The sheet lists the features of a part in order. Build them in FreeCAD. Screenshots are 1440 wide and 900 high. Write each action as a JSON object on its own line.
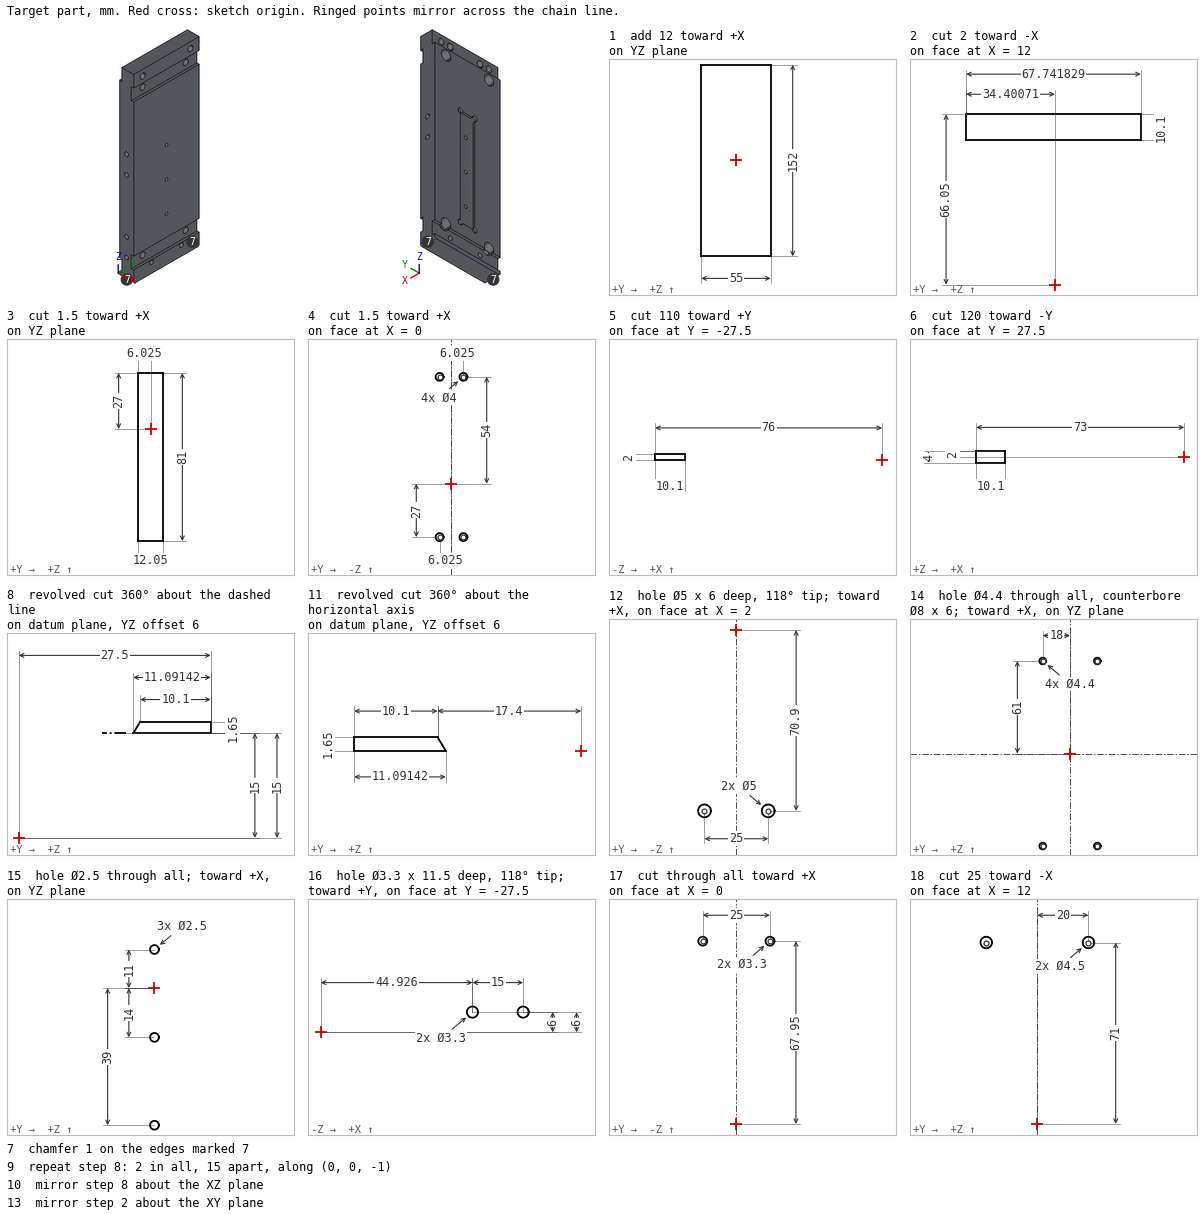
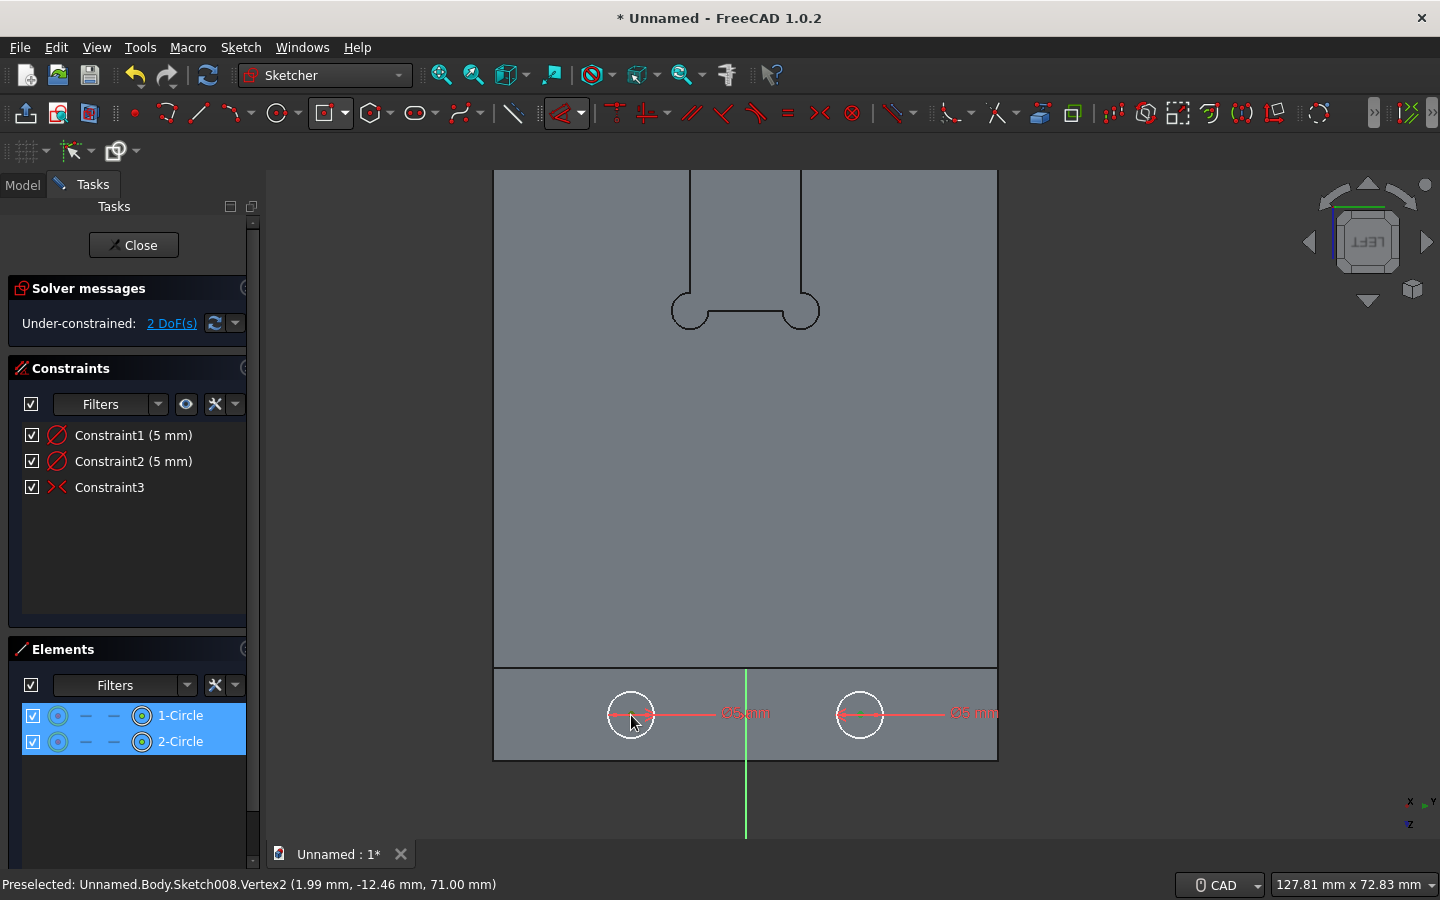
{"action": "key", "text": "l"}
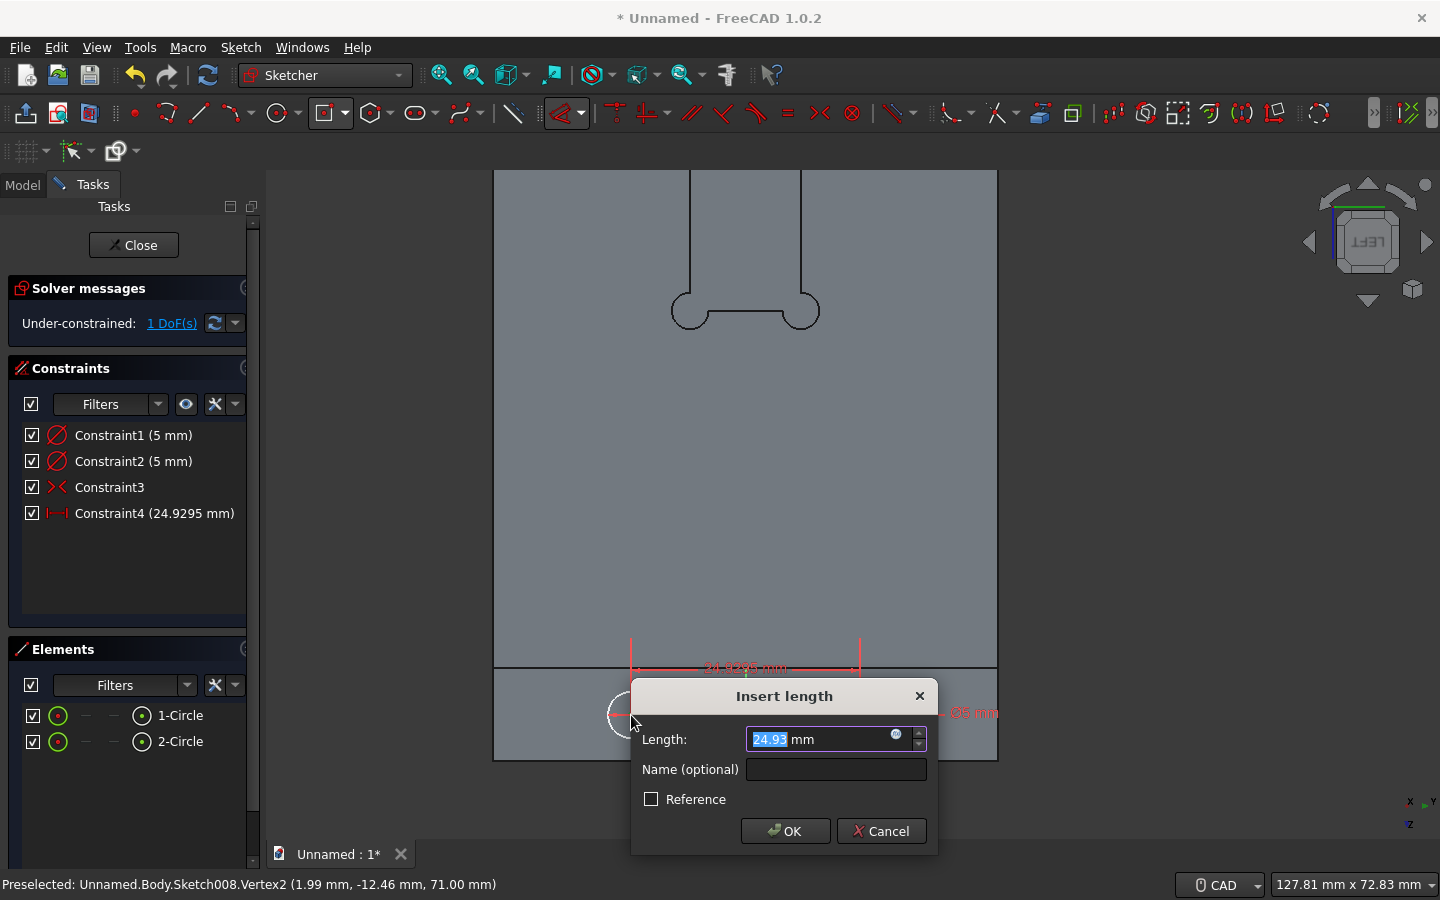
{"action": "type", "text": "25"}
{"action": "key", "text": "Return"}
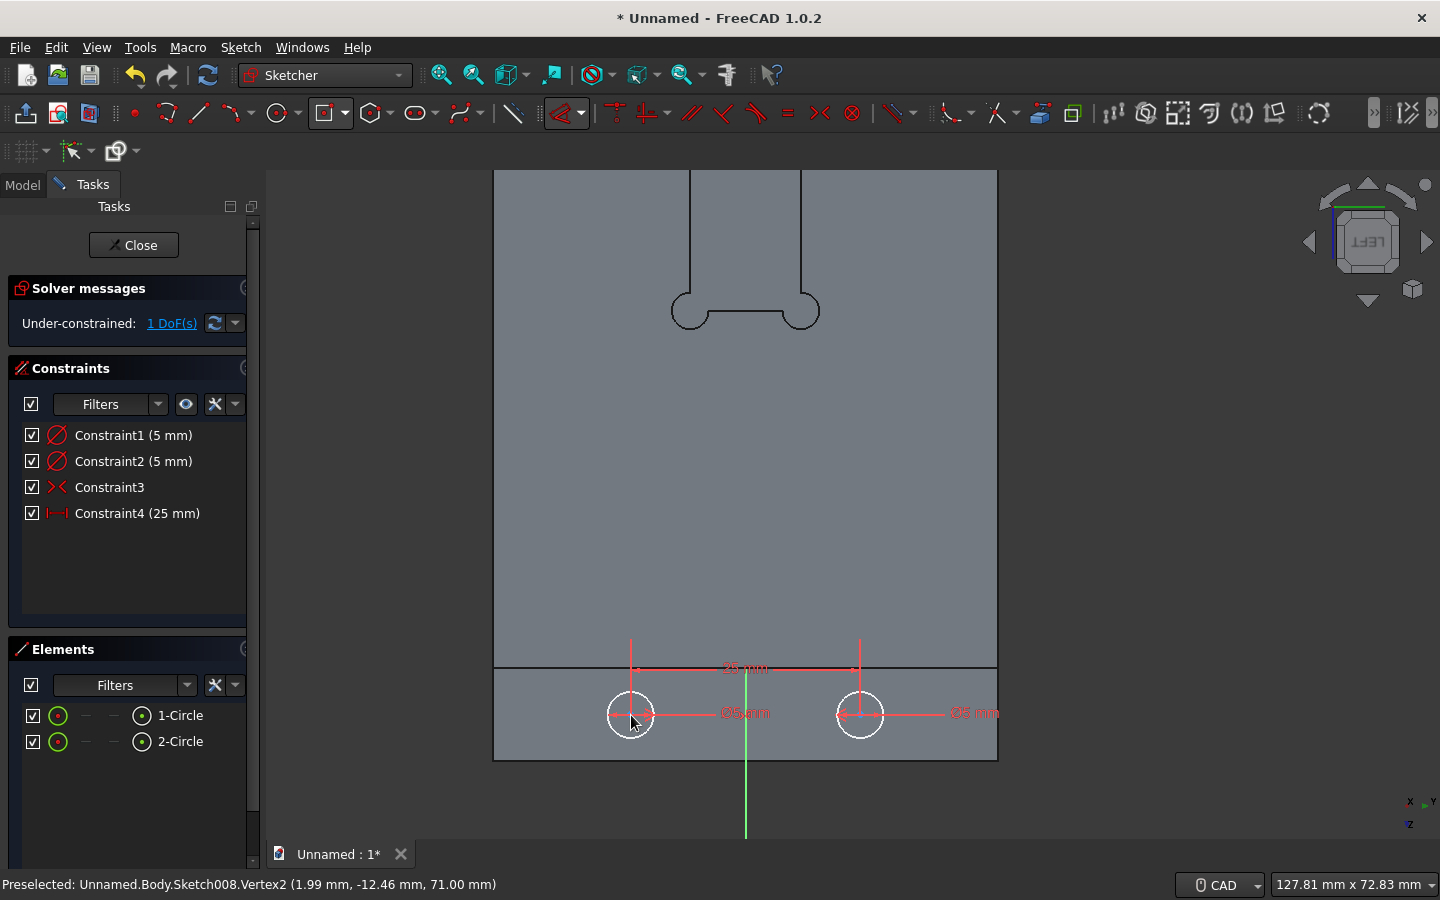
{"action": "left_click", "coordinate": [860, 715]}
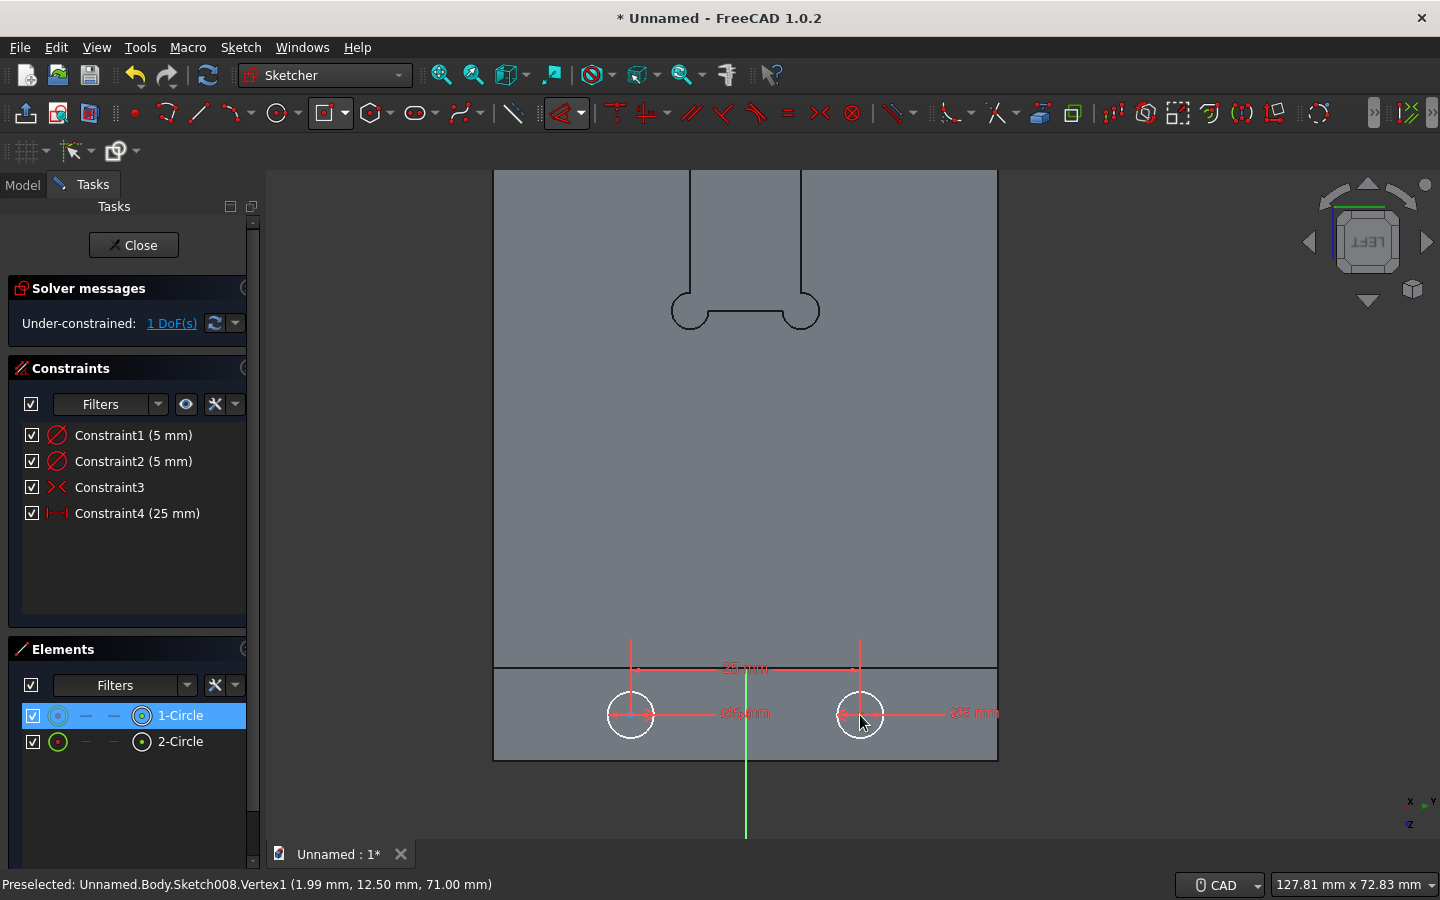
{"action": "key", "text": "i"}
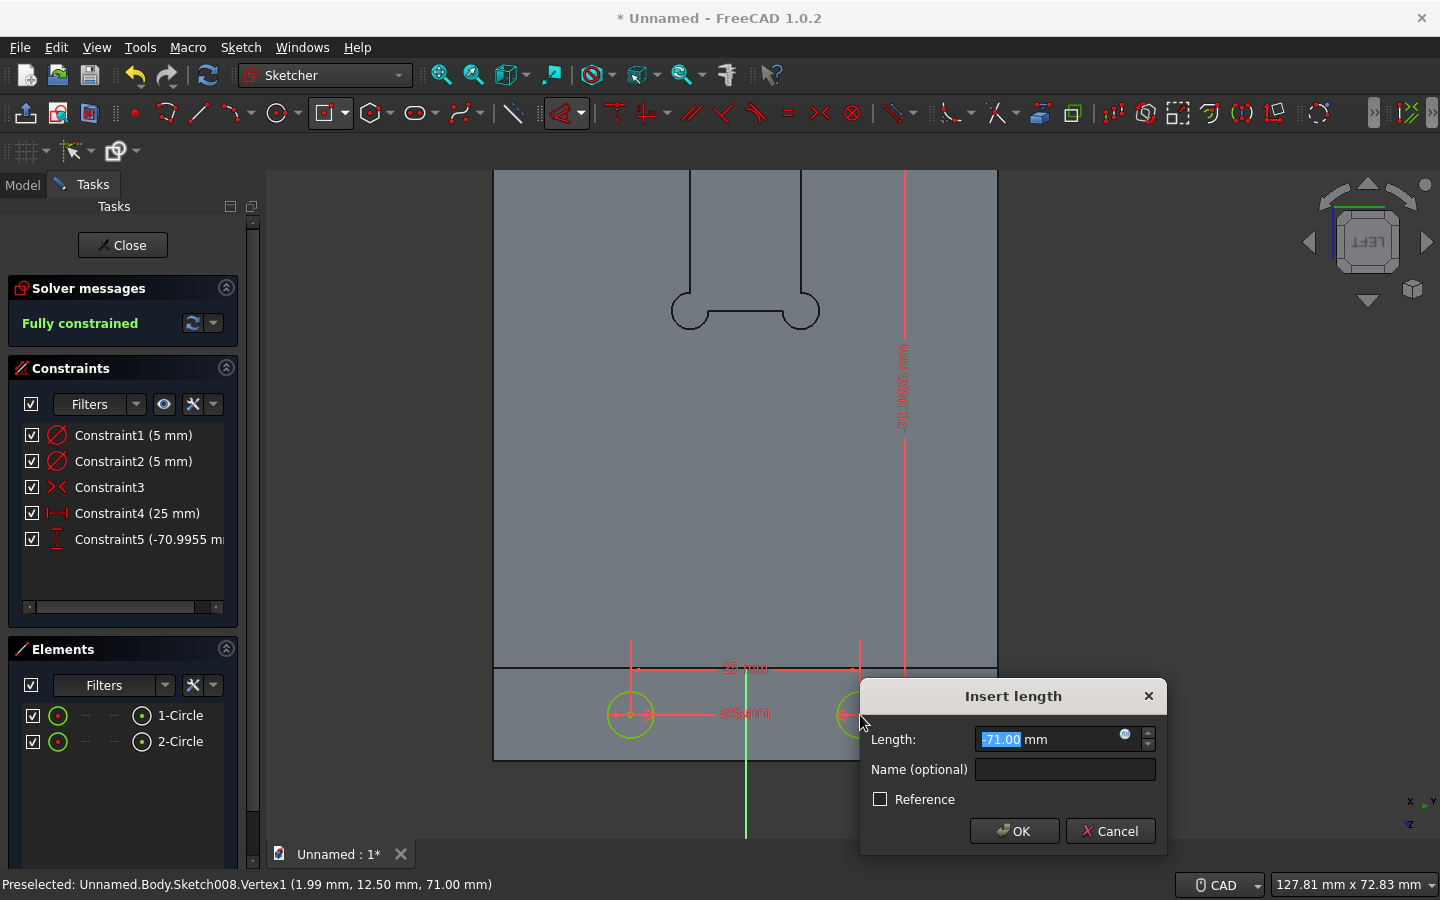
{"action": "type", "text": "-70.9"}
{"action": "key", "text": "Return"}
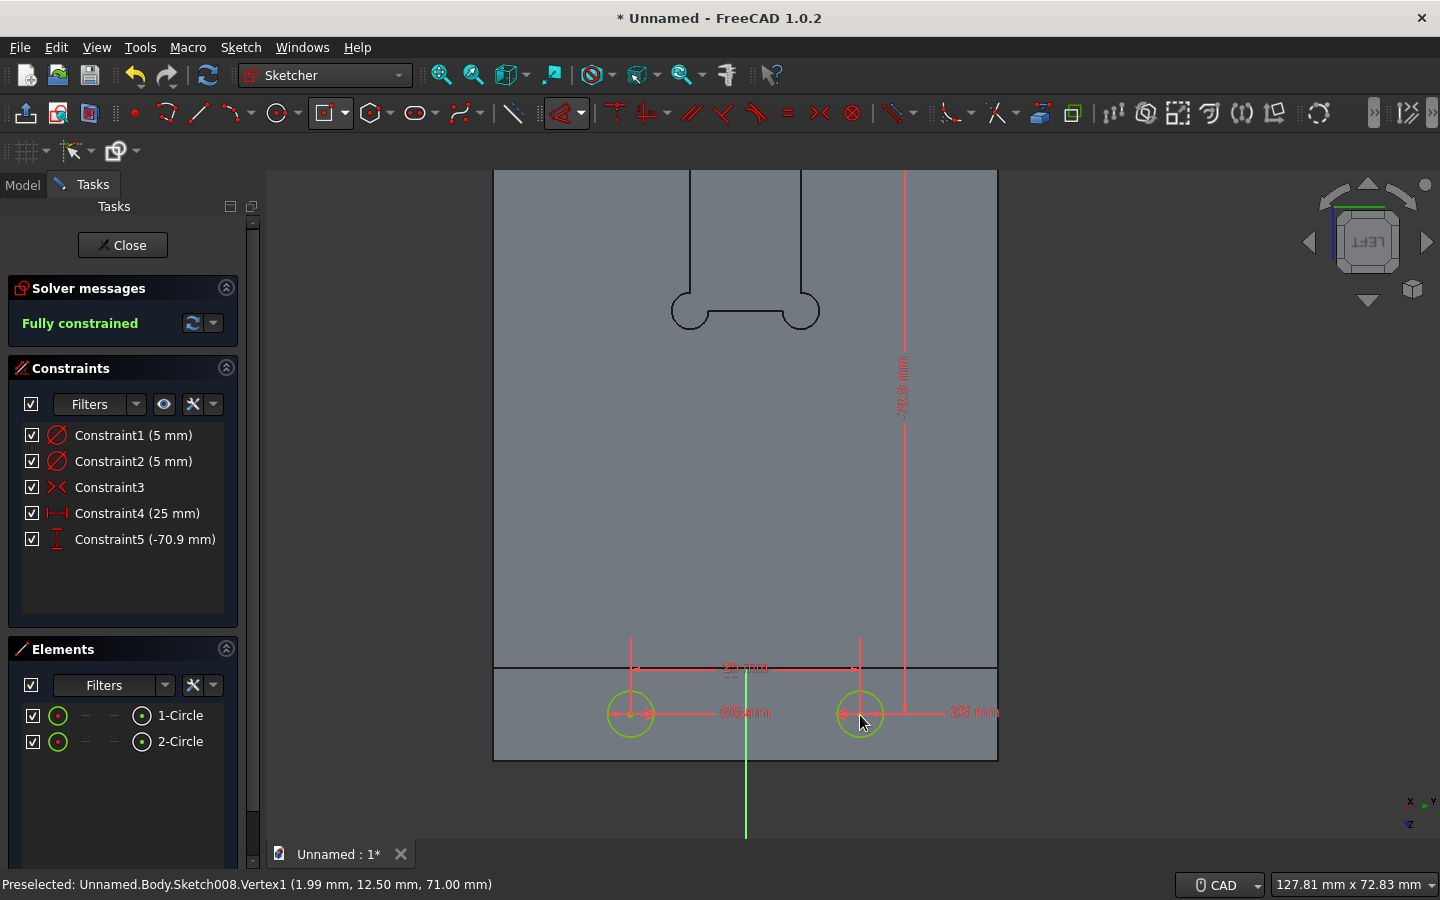
{"action": "left_click", "coordinate": [123, 245]}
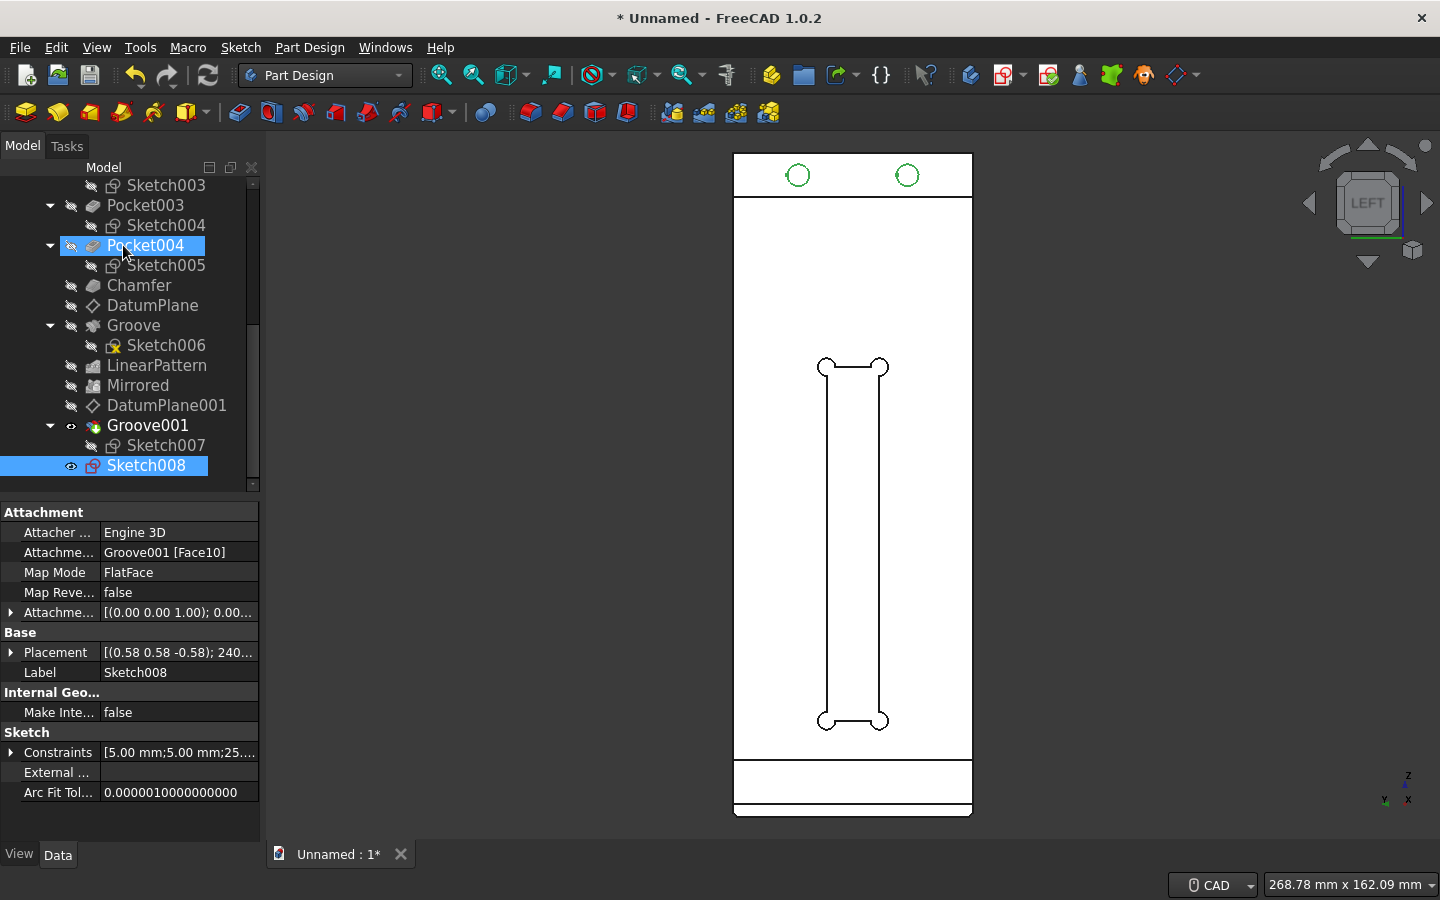
{"action": "left_click", "coordinate": [272, 112]}